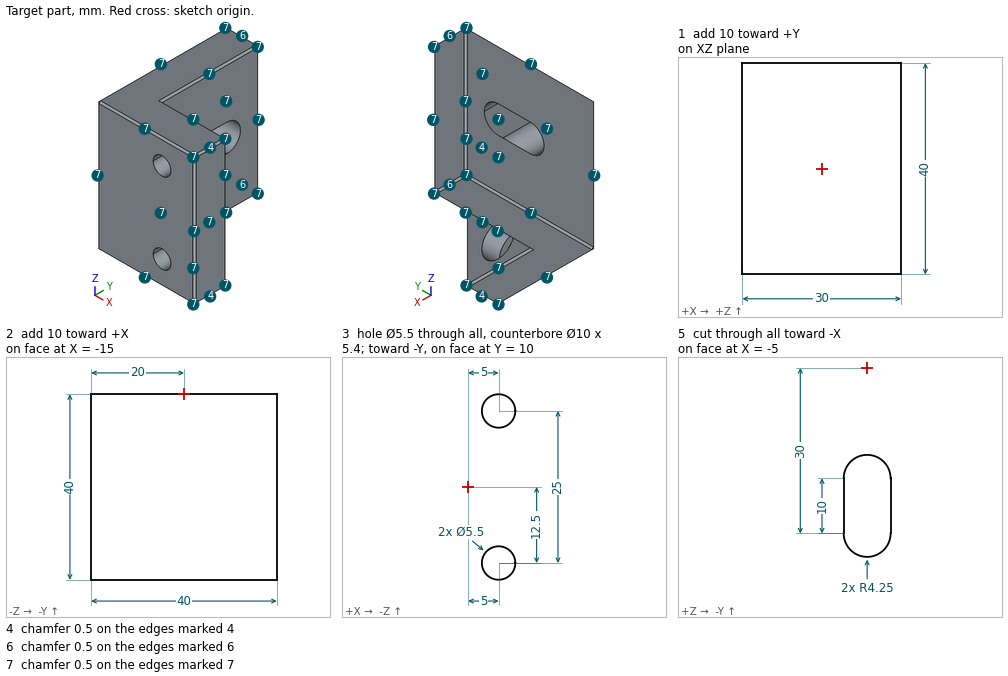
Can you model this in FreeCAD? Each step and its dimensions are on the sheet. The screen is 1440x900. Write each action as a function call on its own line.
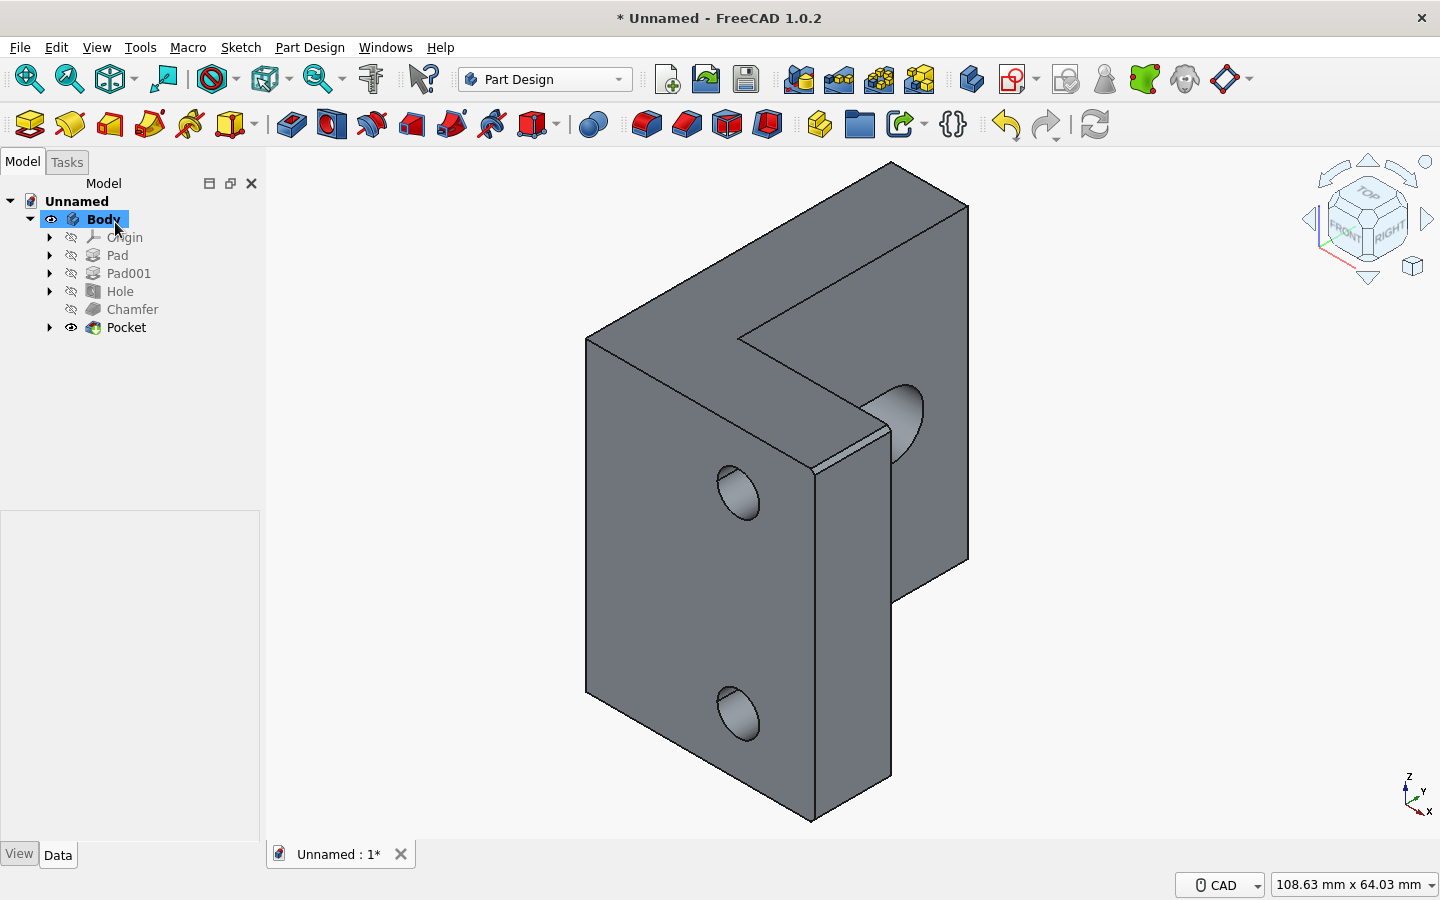
key(2)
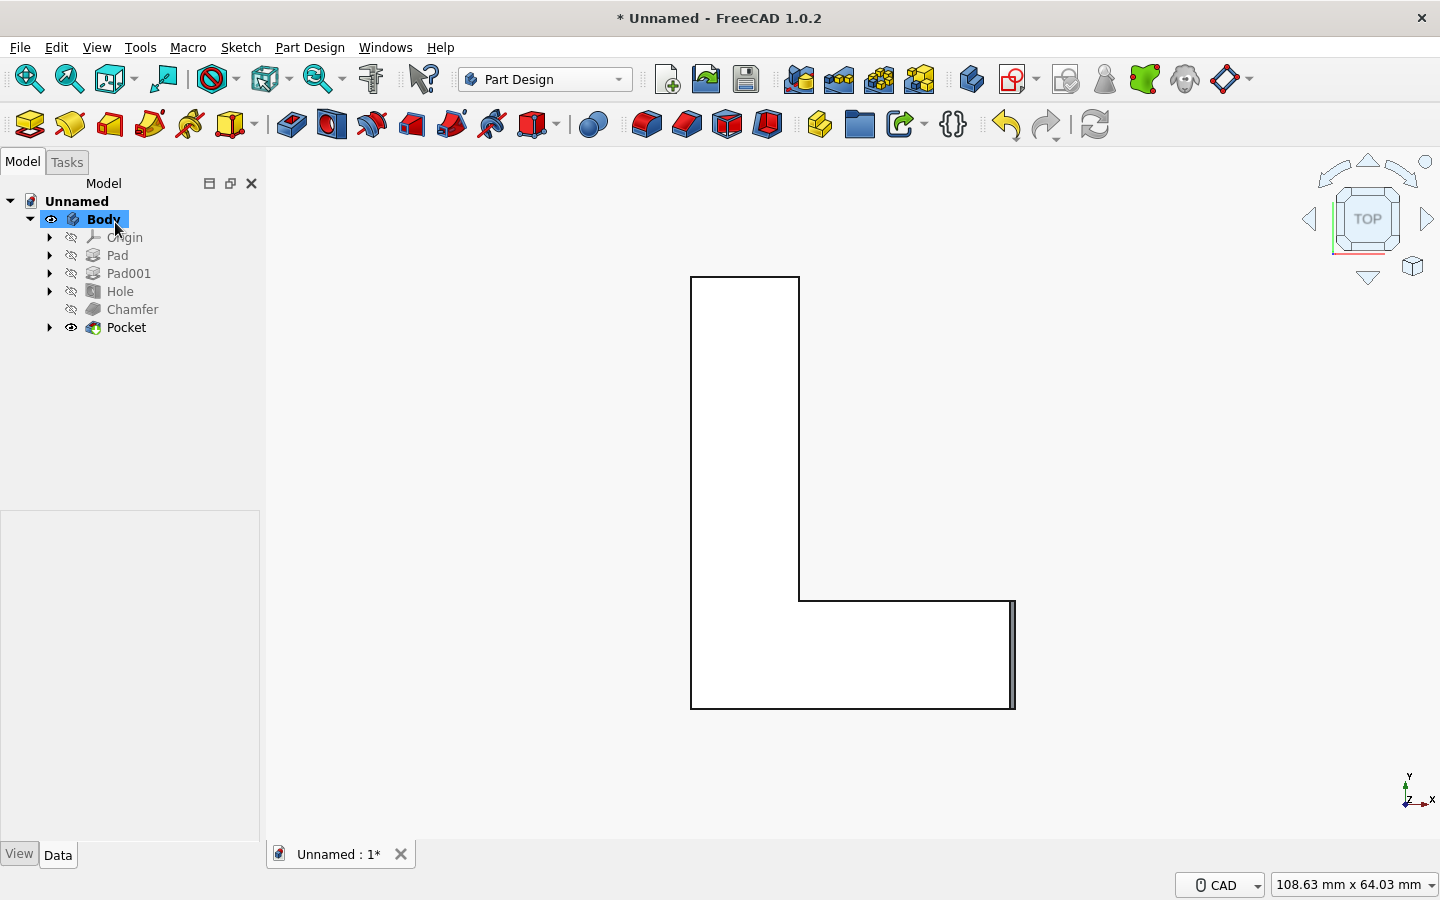
click(745, 276)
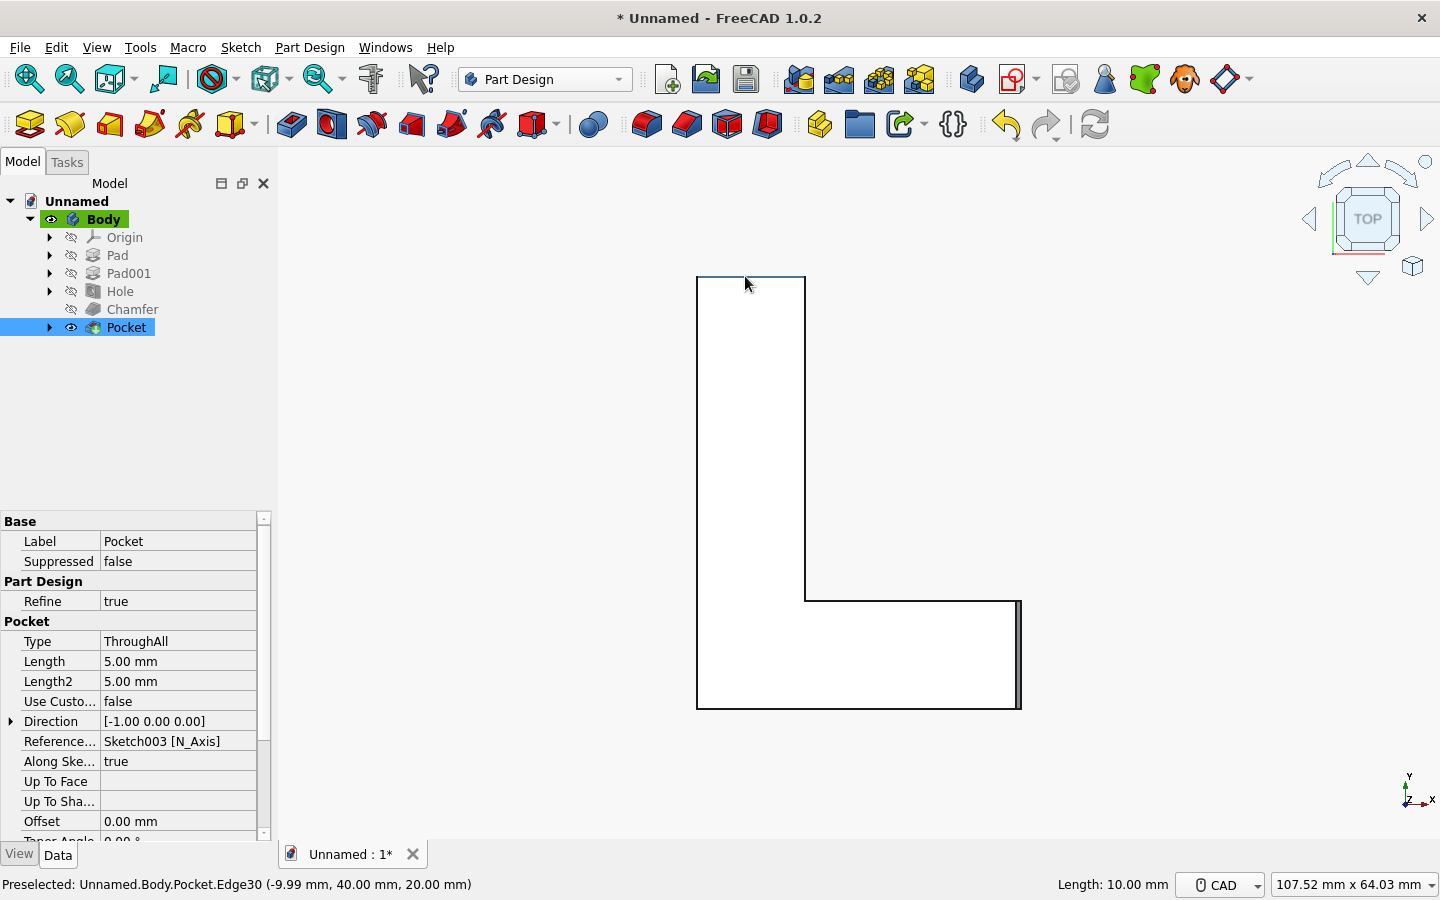
key(1)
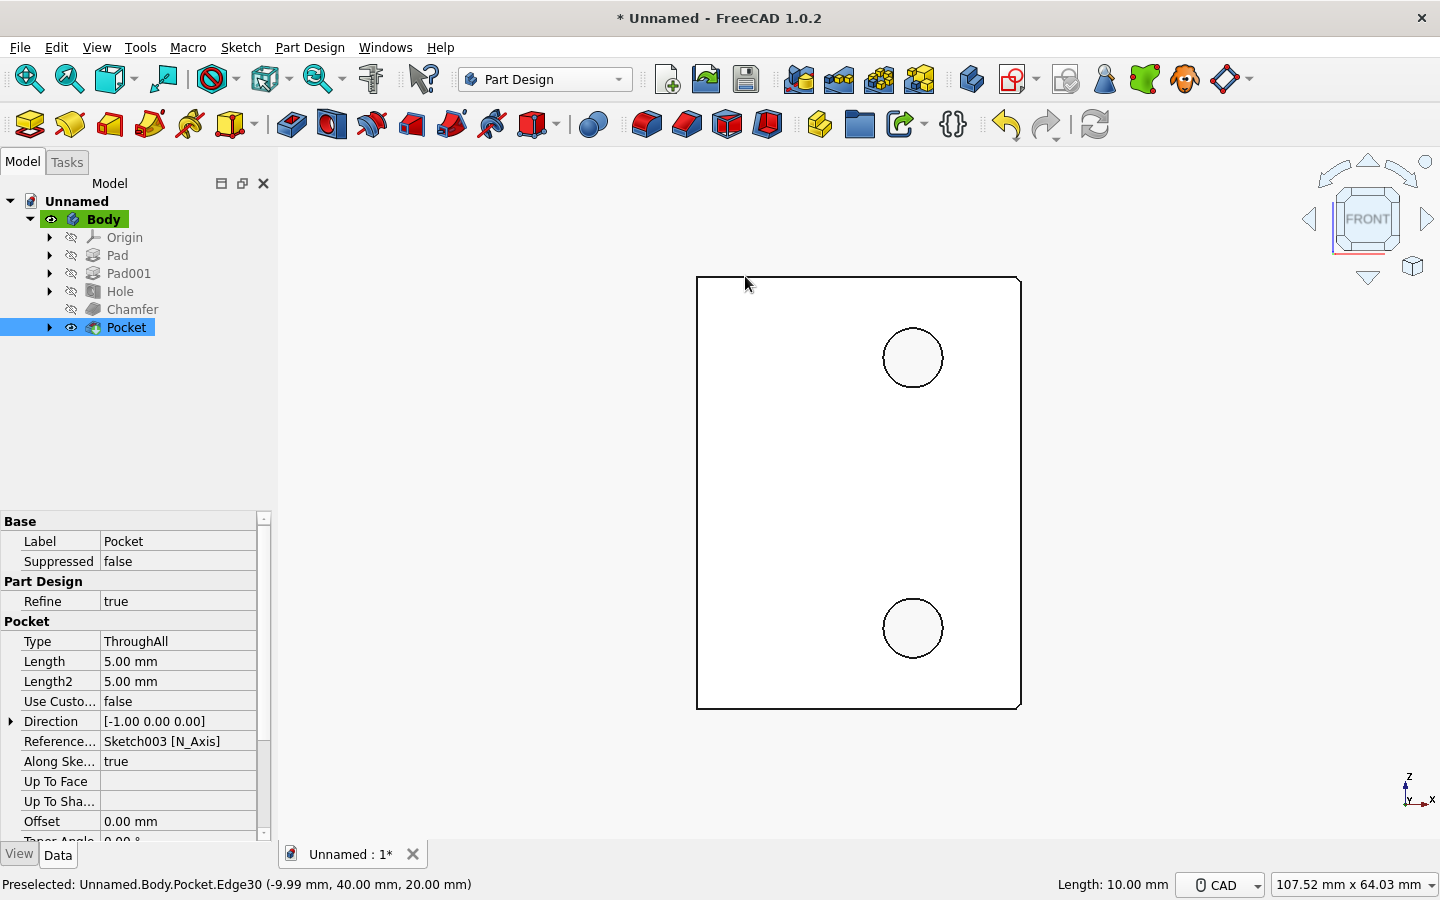
key(3)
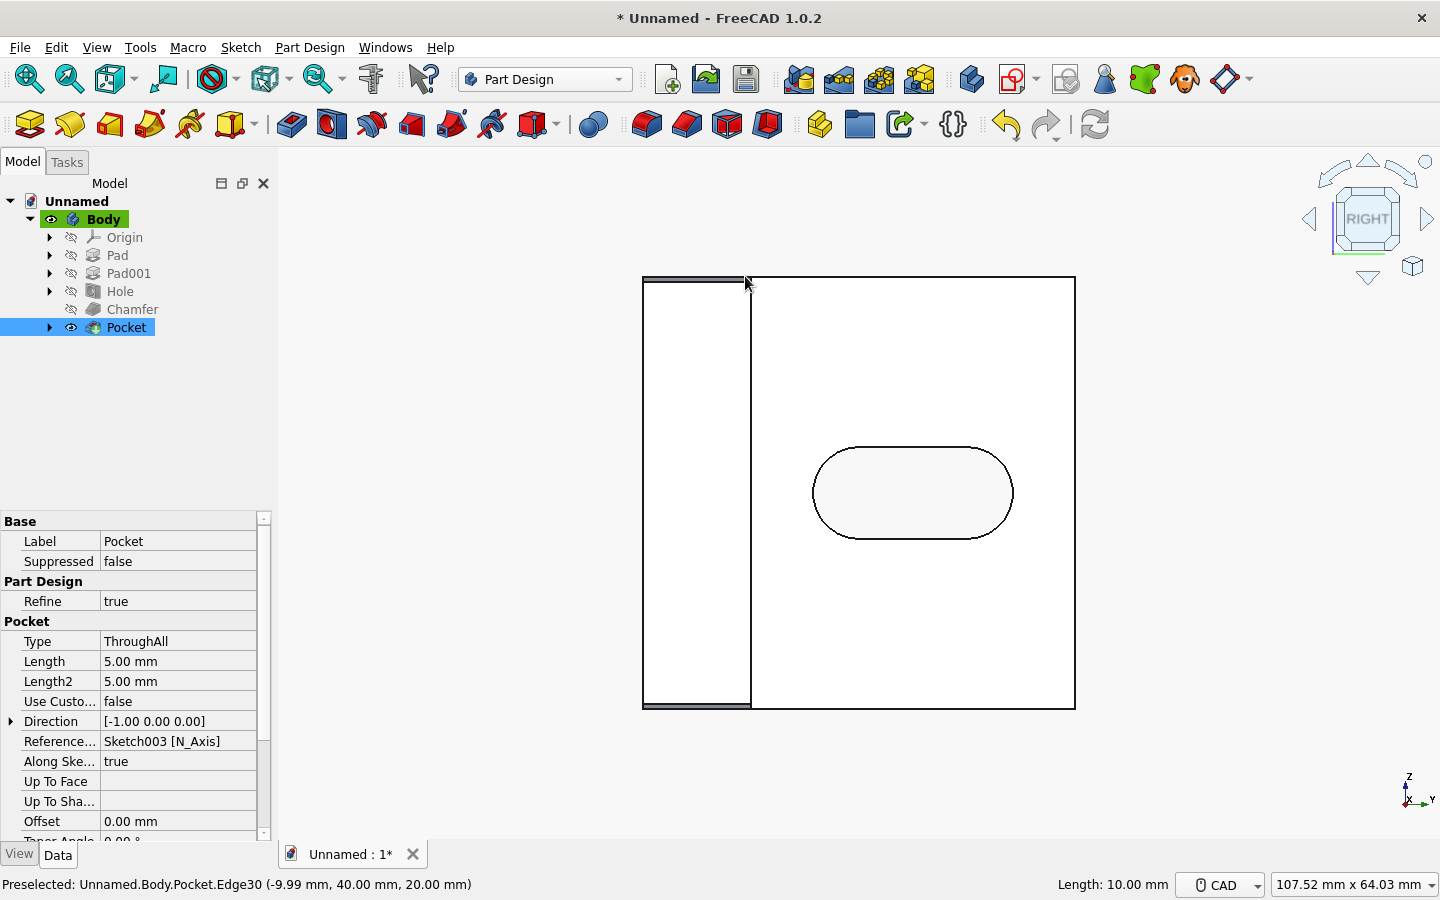
key(5)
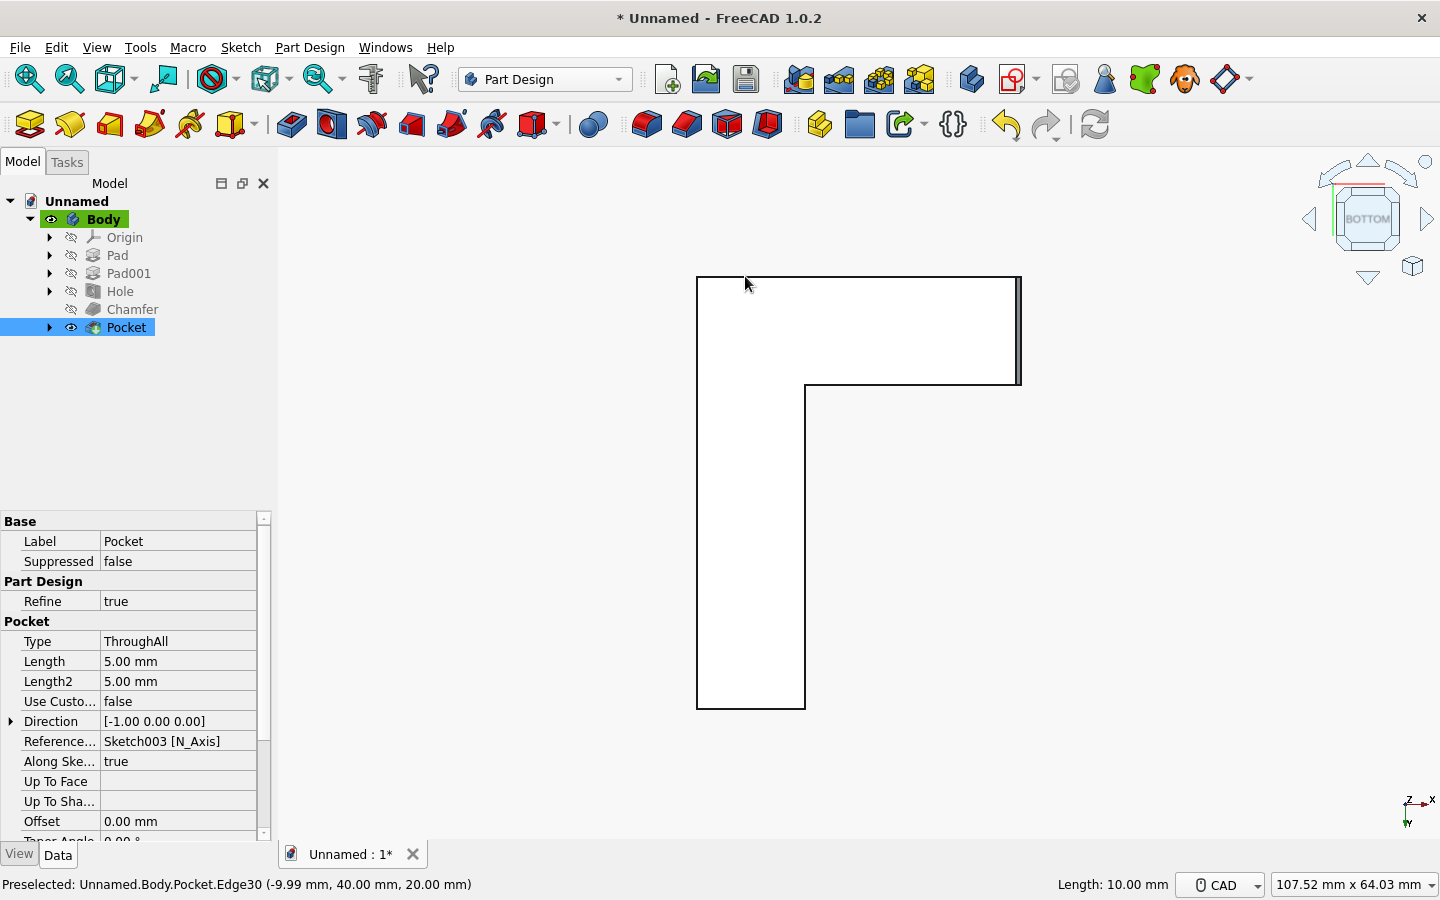
key(4)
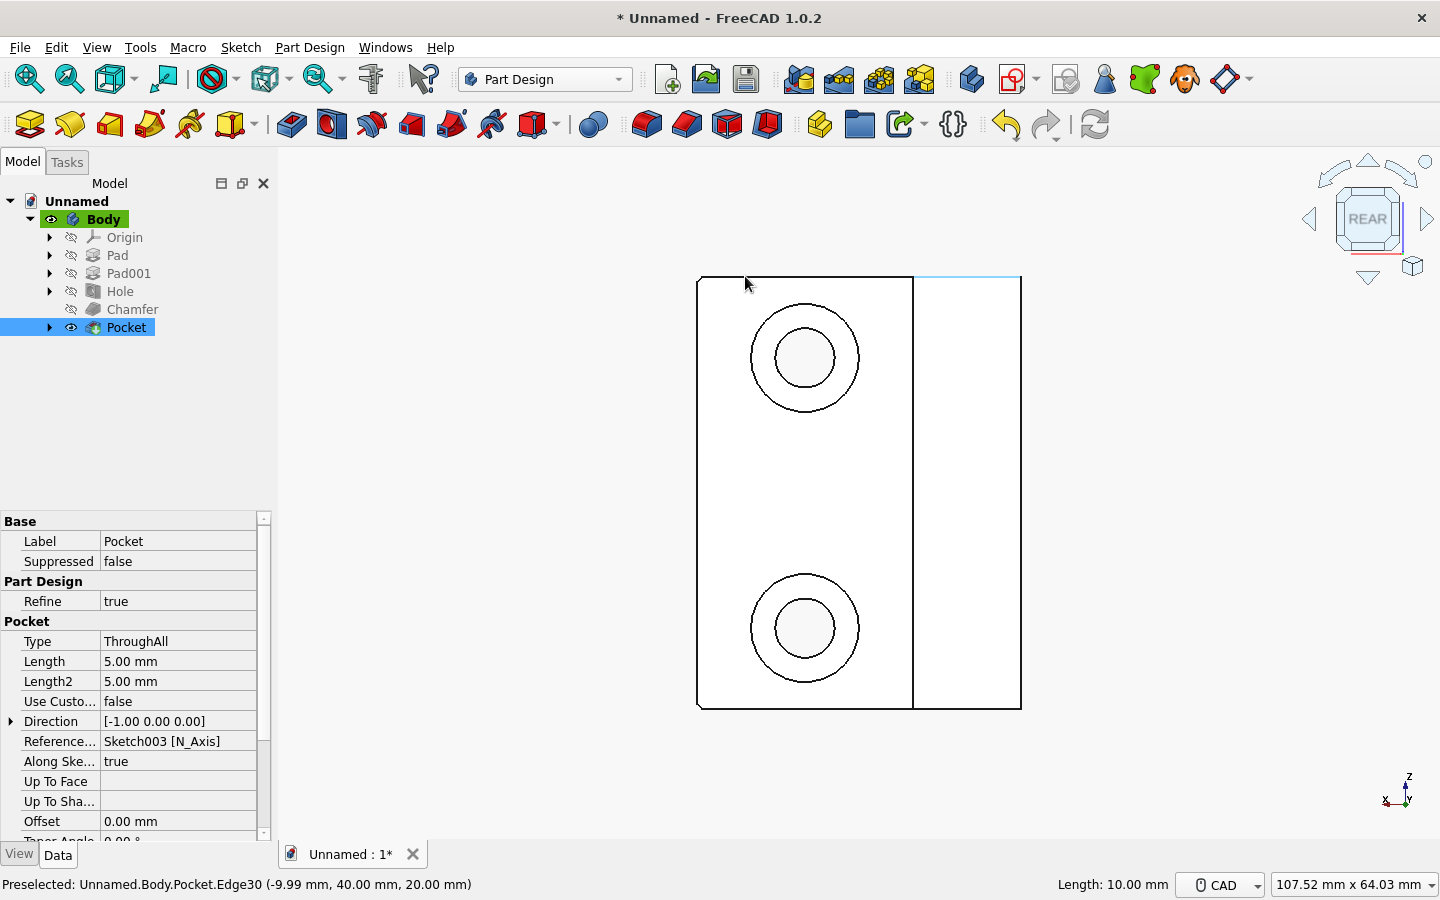
click(967, 708, ctrl)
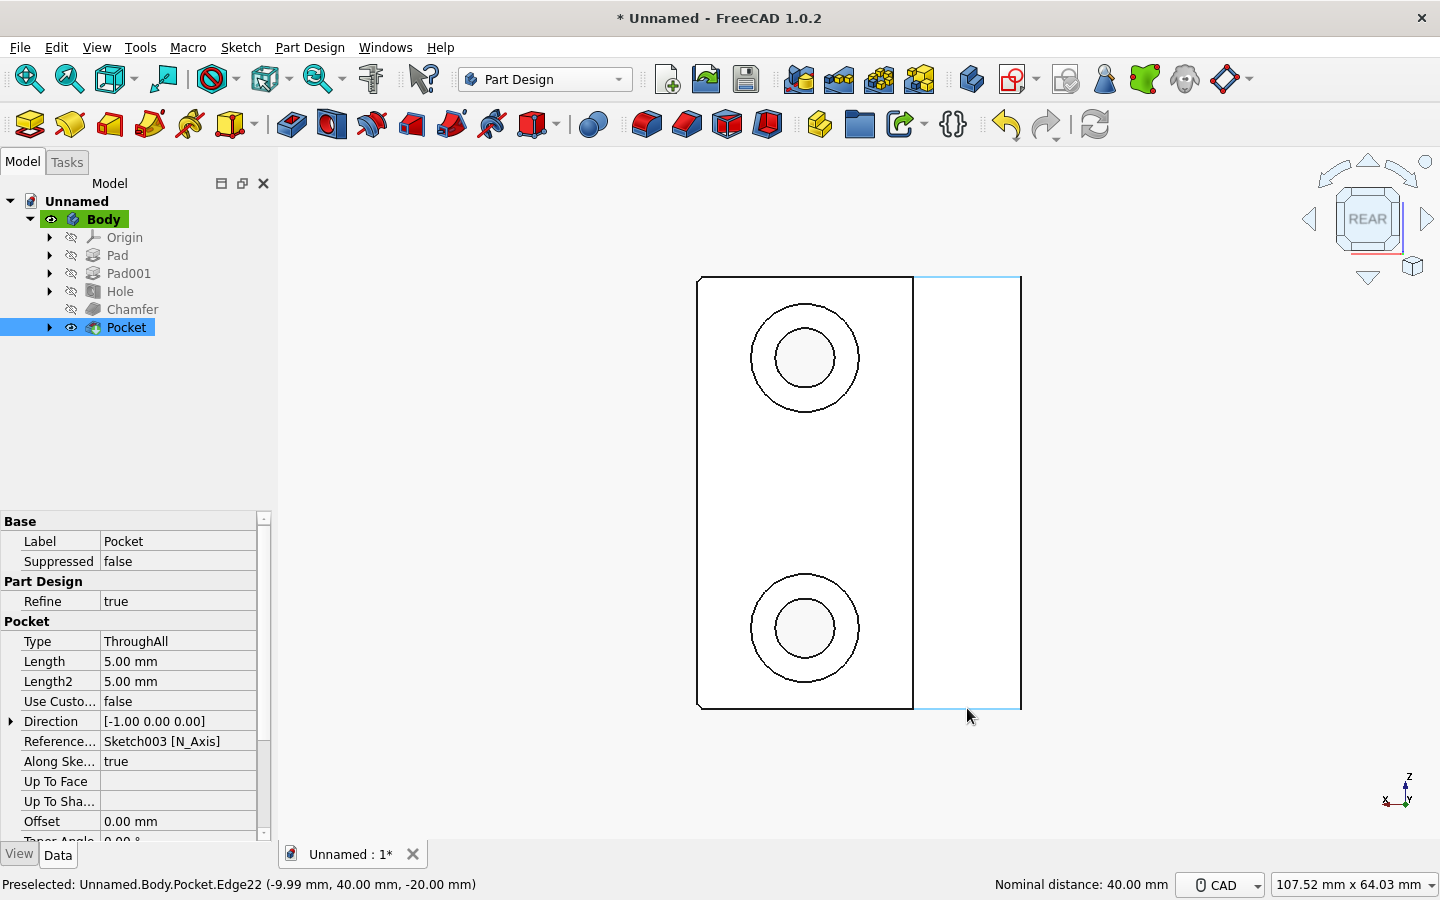
click(688, 124)